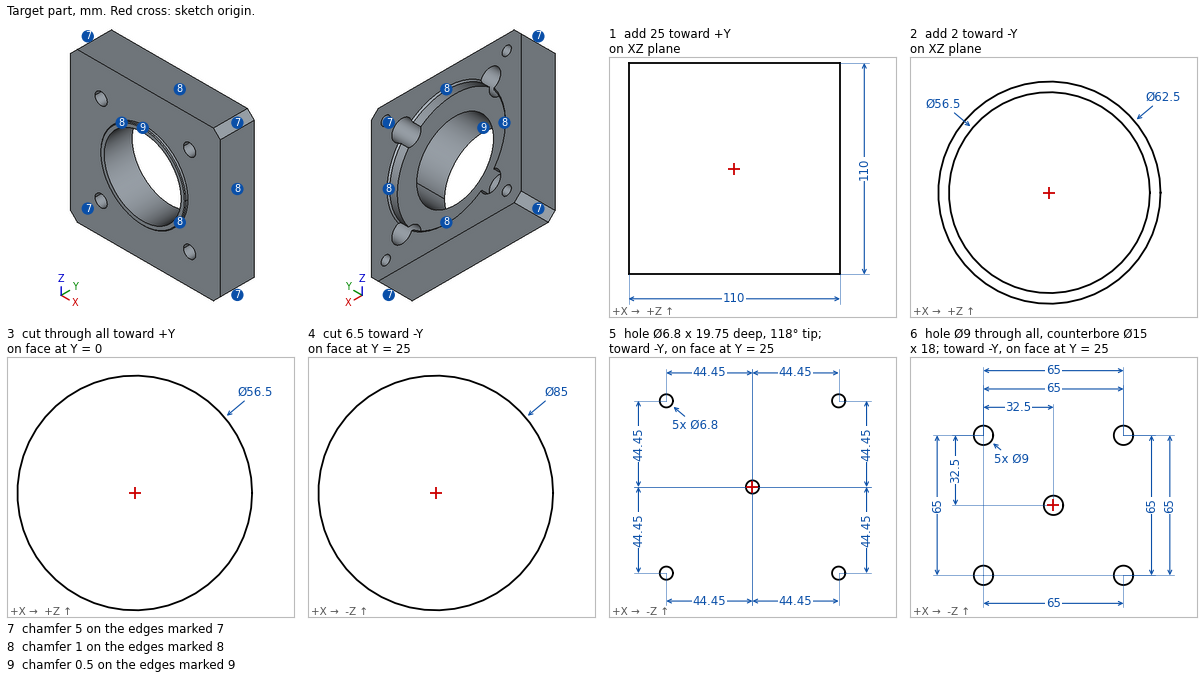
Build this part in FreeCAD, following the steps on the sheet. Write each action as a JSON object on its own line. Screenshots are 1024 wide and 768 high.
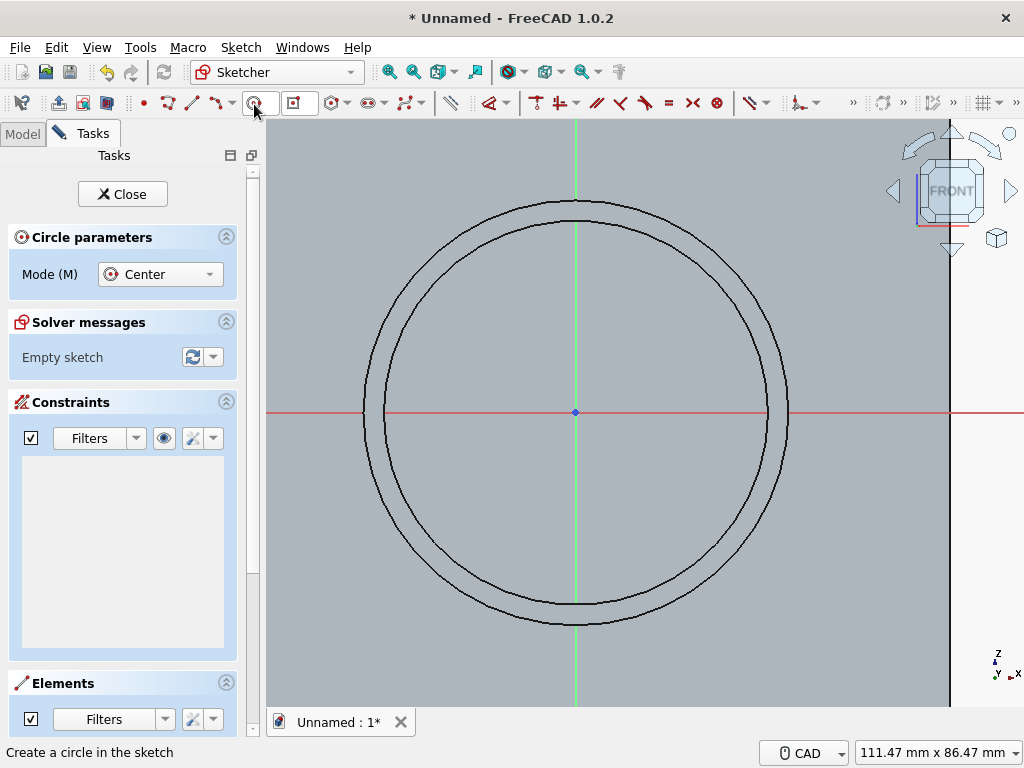
{"action": "left_click", "coordinate": [576, 413]}
{"action": "left_click", "coordinate": [712, 277]}
{"action": "key", "text": "Escape"}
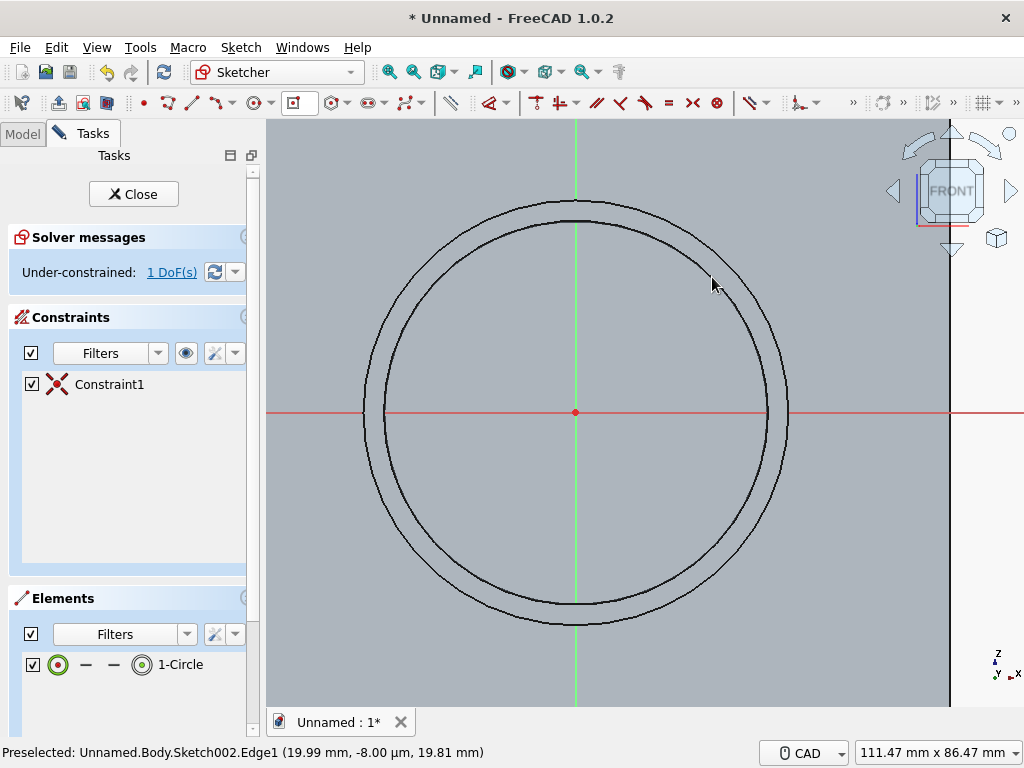
{"action": "left_click", "coordinate": [490, 104]}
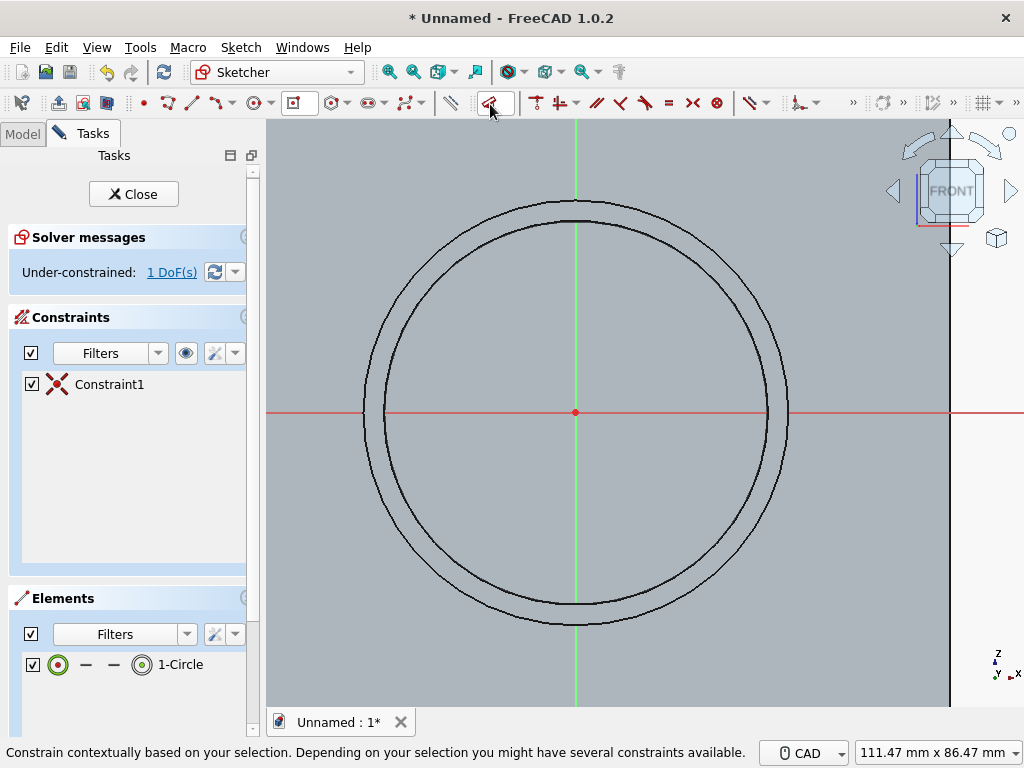
{"action": "left_click", "coordinate": [711, 277]}
{"action": "left_click", "coordinate": [734, 254]}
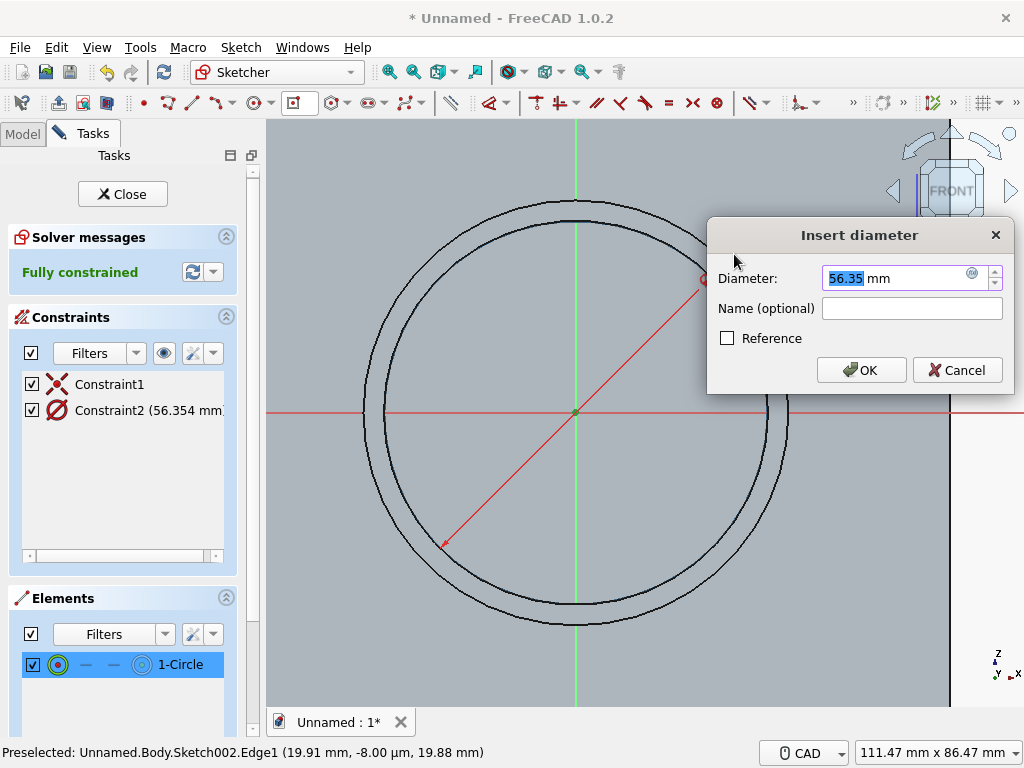
{"action": "type", "text": "56.5"}
{"action": "key", "text": "Return"}
{"action": "key", "text": "Escape"}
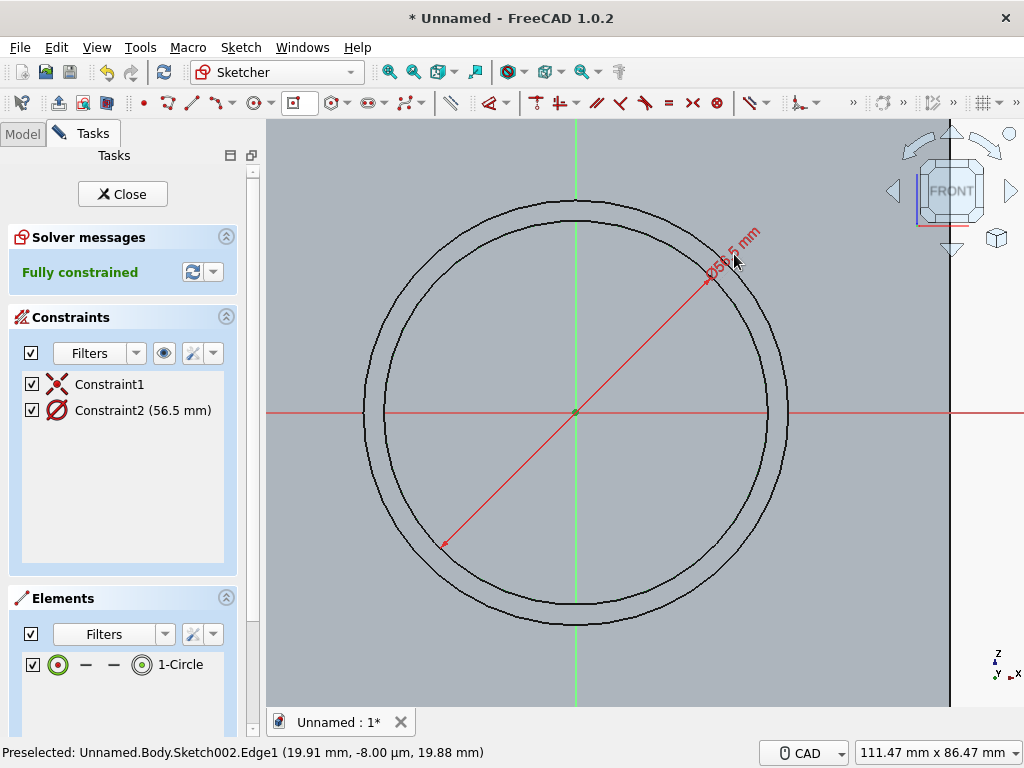
{"action": "left_click", "coordinate": [123, 194]}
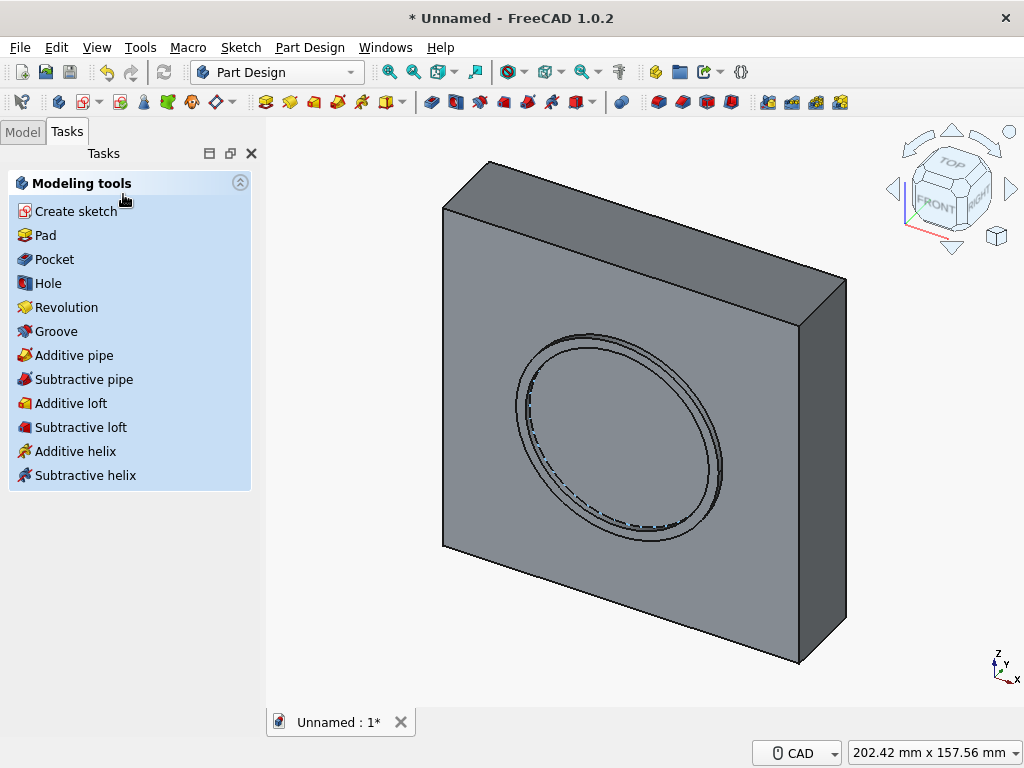
{"action": "left_click", "coordinate": [432, 102]}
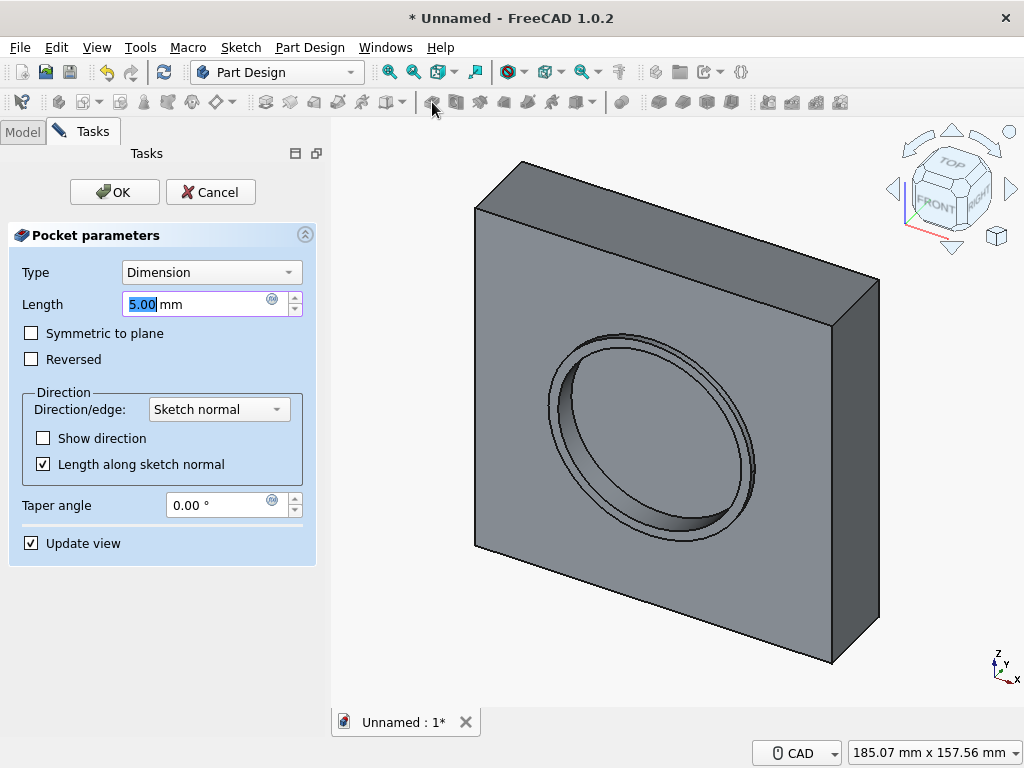
{"action": "left_click", "coordinate": [212, 272]}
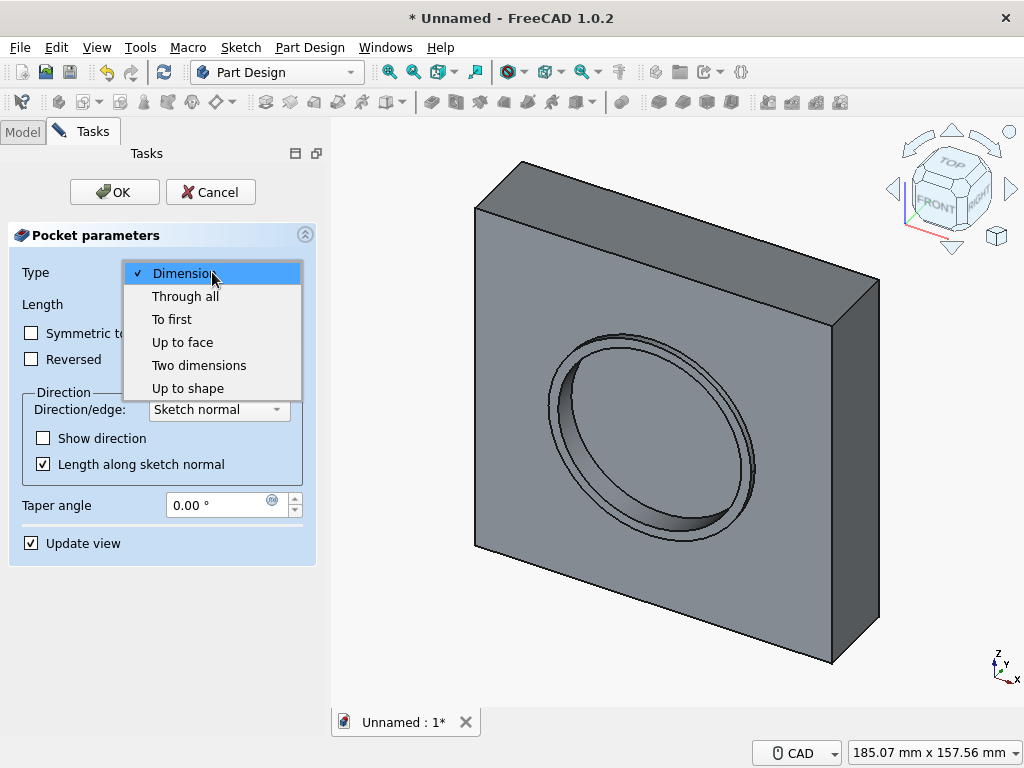
{"action": "left_click", "coordinate": [212, 296]}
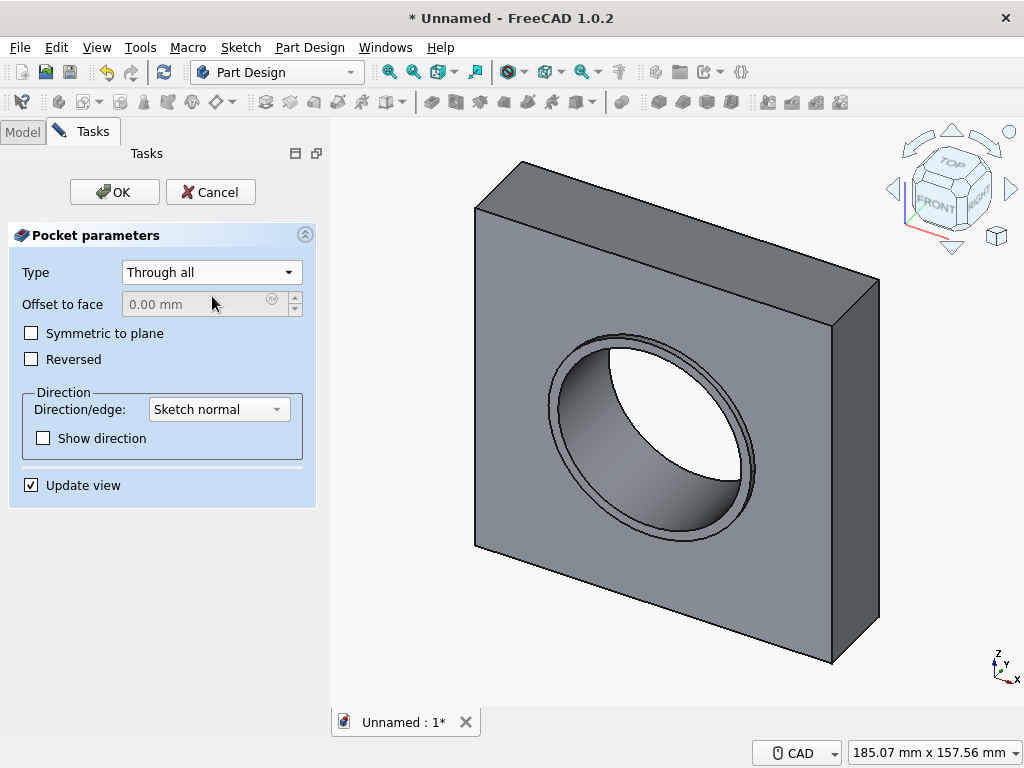
{"action": "left_click", "coordinate": [115, 192]}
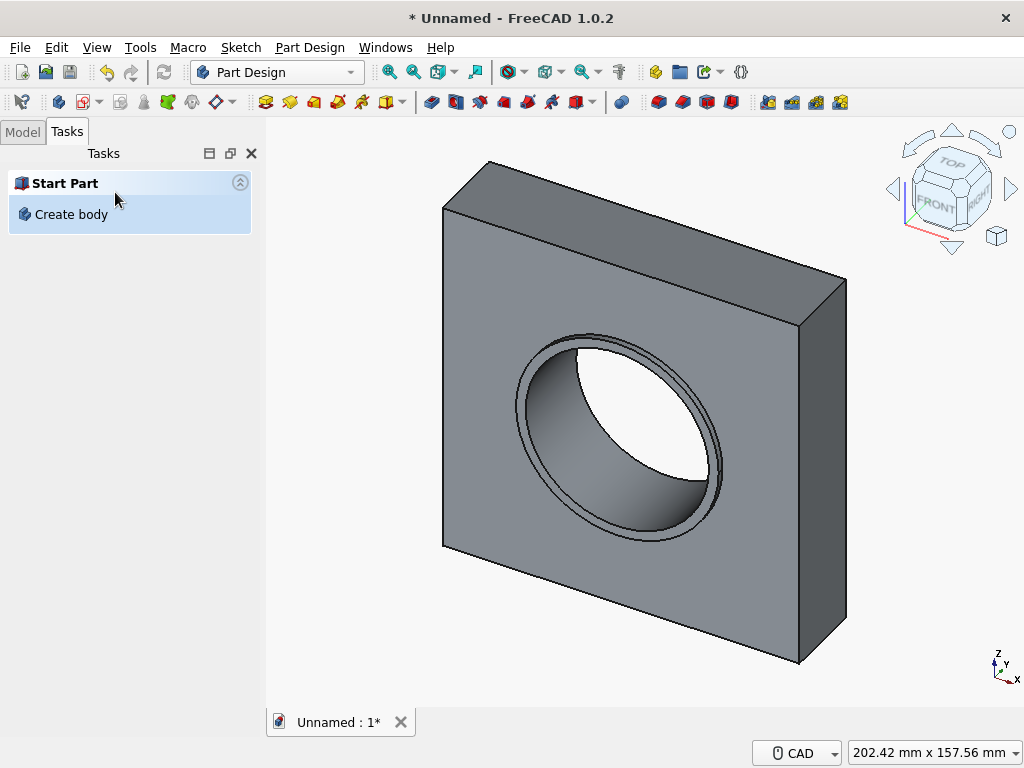
{"action": "key", "text": "4"}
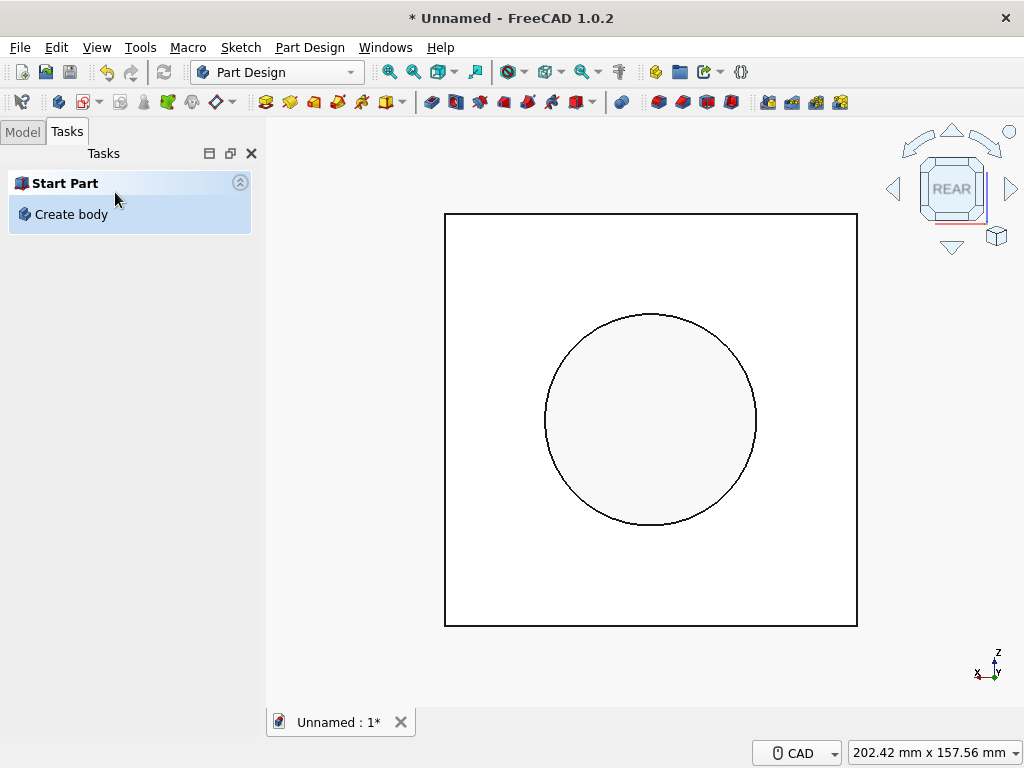
{"action": "left_click", "coordinate": [533, 301]}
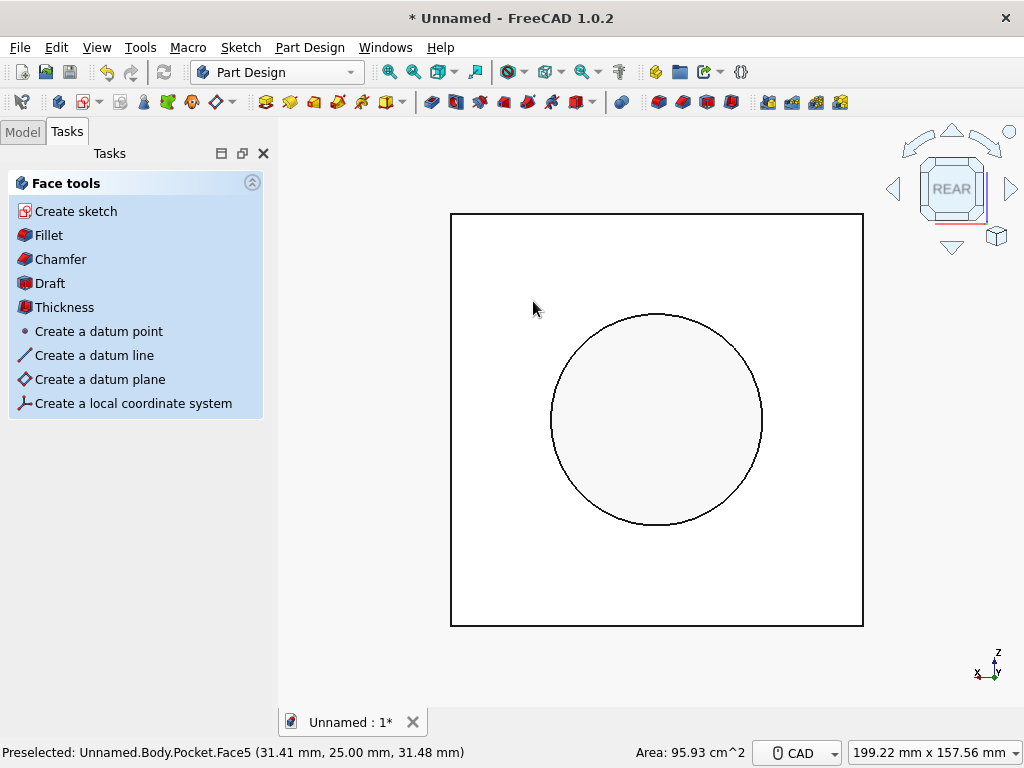
{"action": "left_click", "coordinate": [84, 102]}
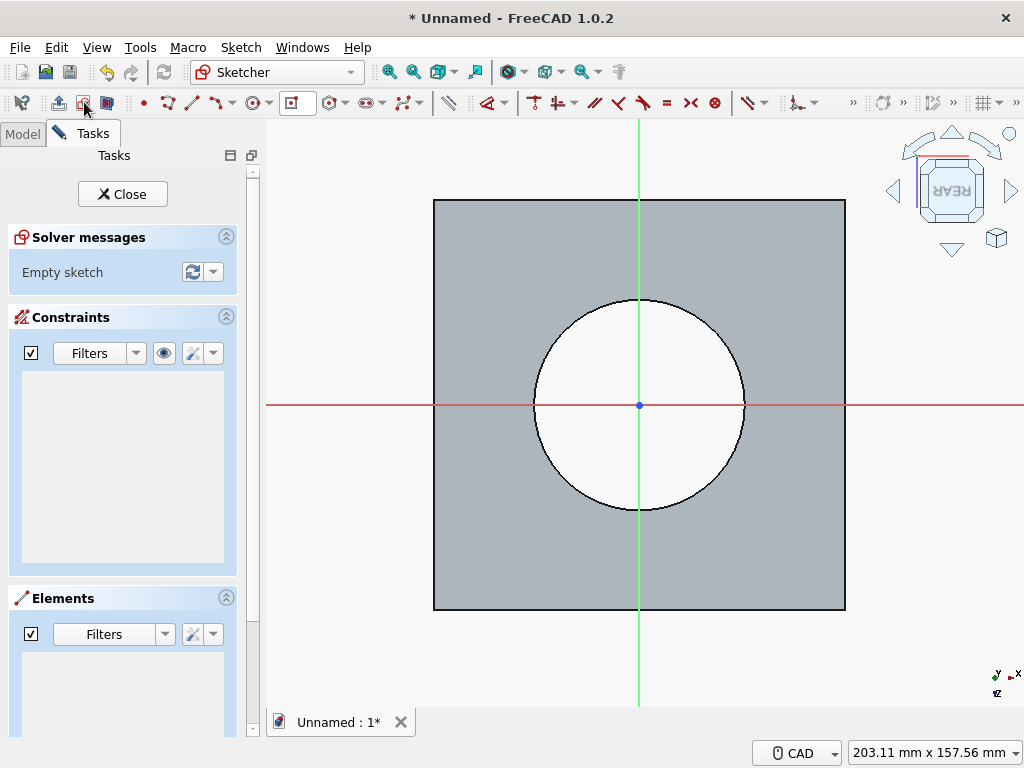
{"action": "left_click", "coordinate": [254, 104]}